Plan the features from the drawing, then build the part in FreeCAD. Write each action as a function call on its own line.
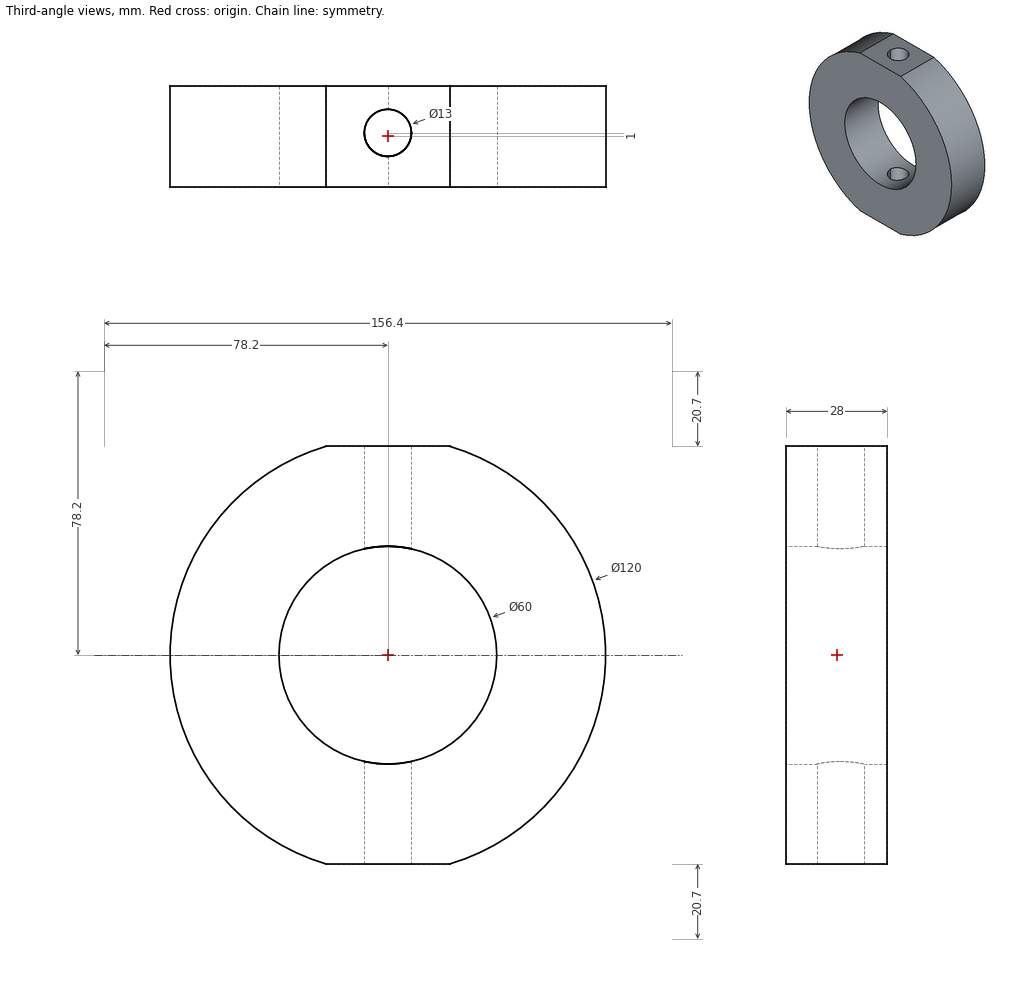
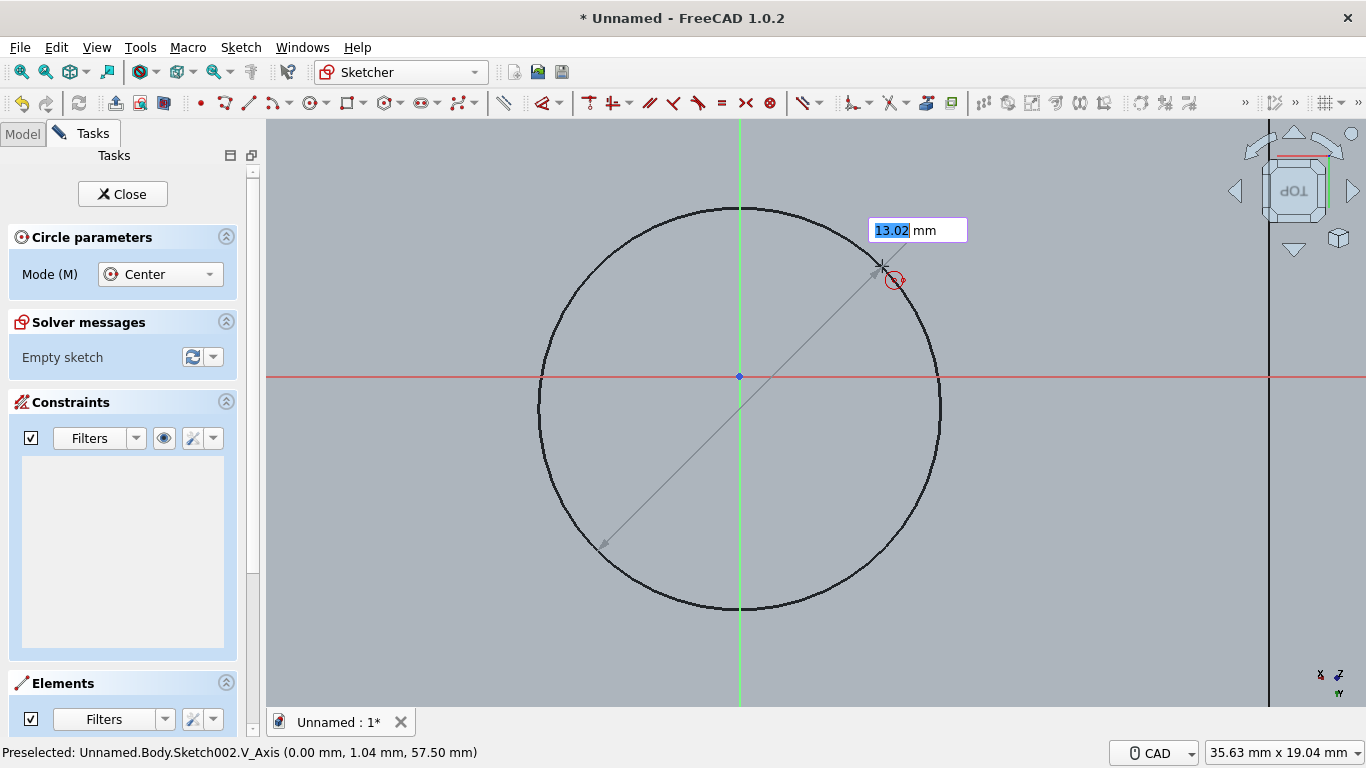
text(13)
key(Return)
key(Escape)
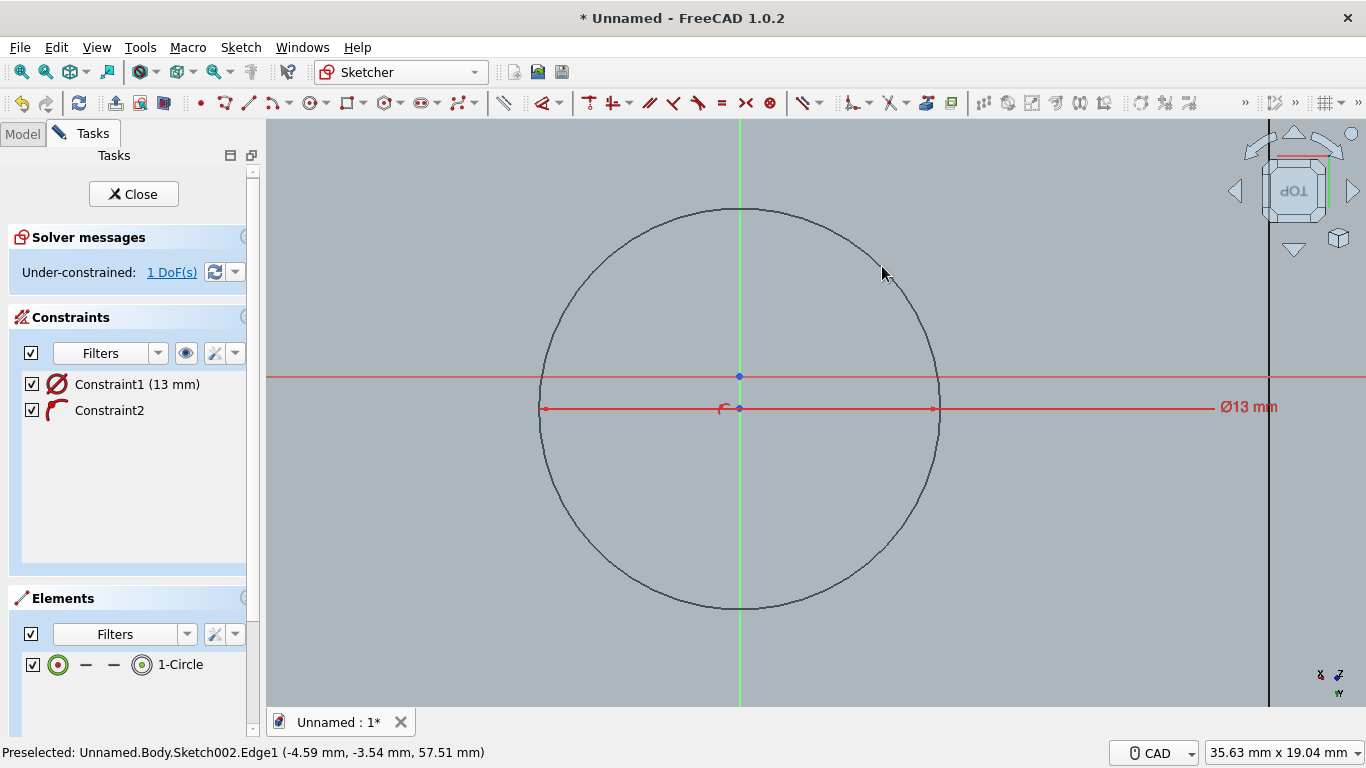
key(d)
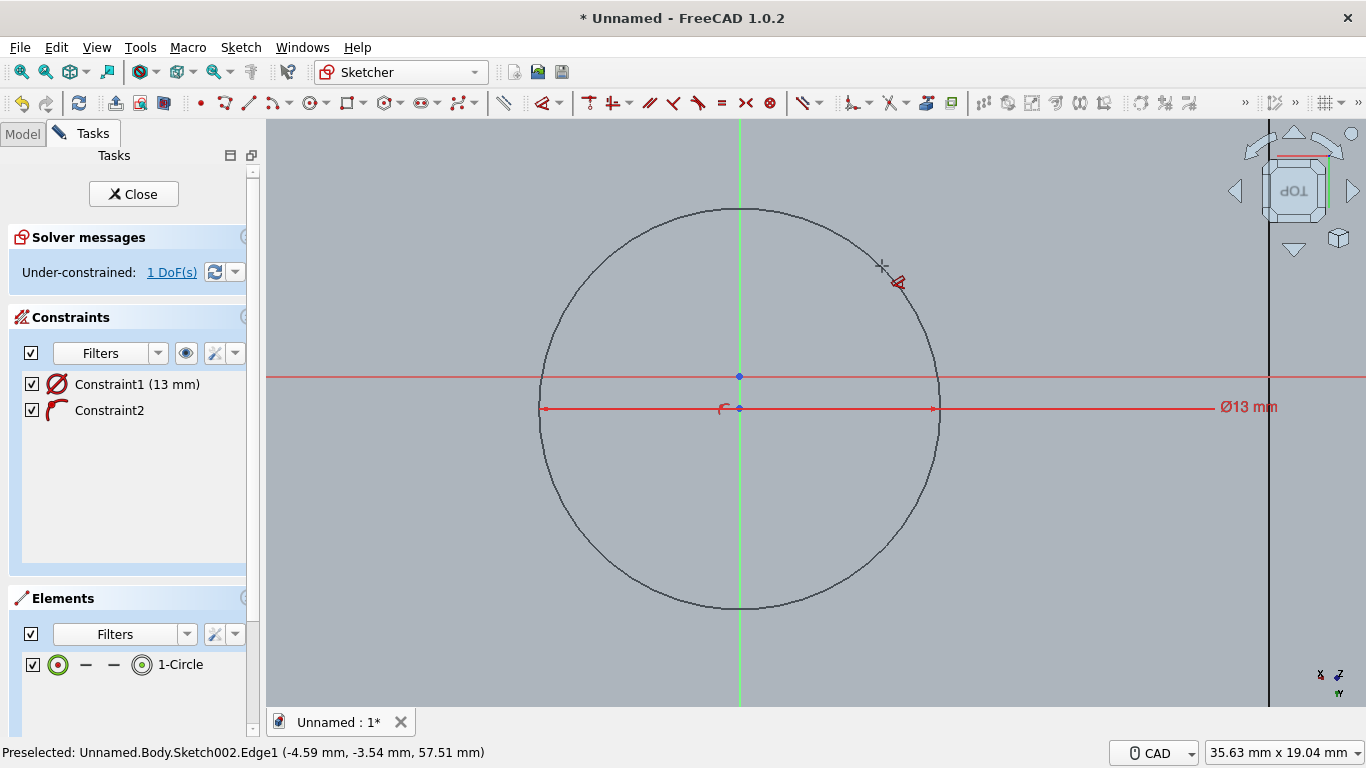
scroll(740, 409, up, 2)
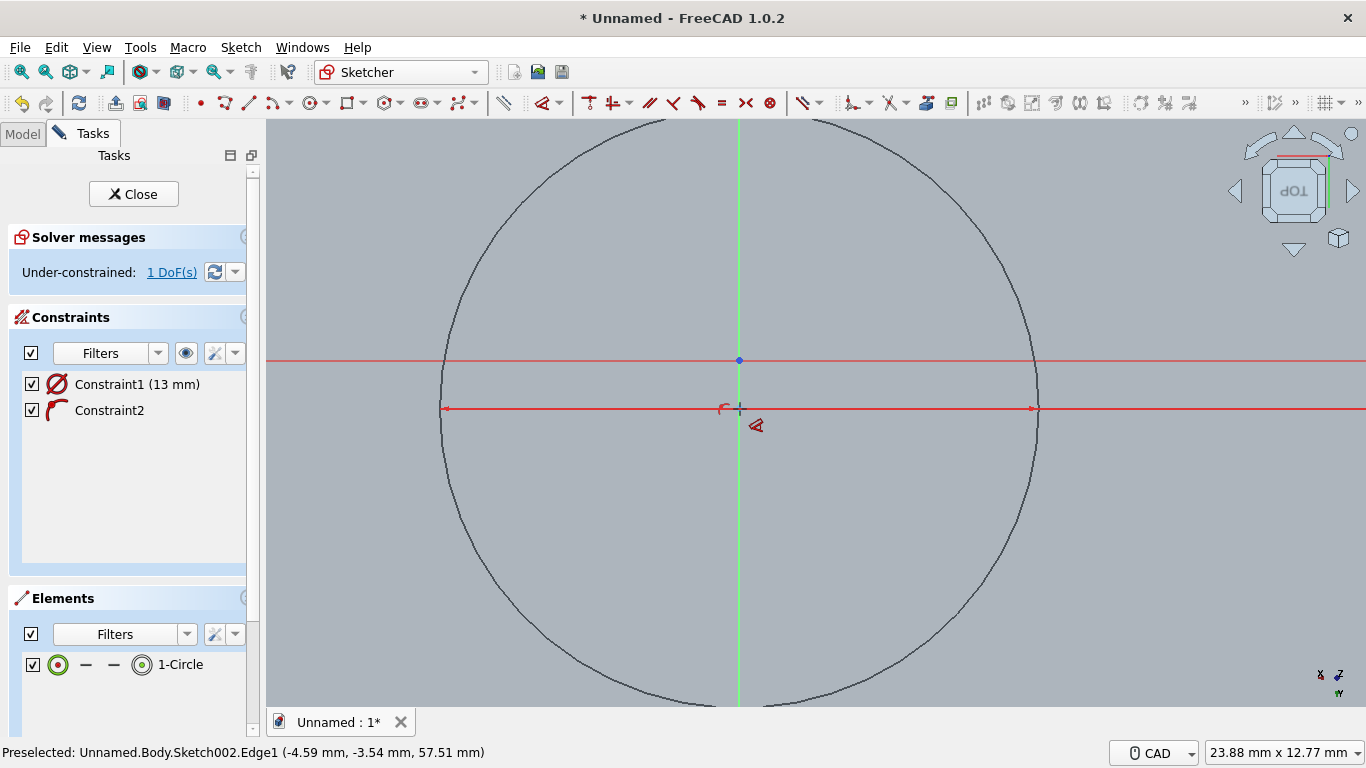
click(739, 409)
click(773, 385)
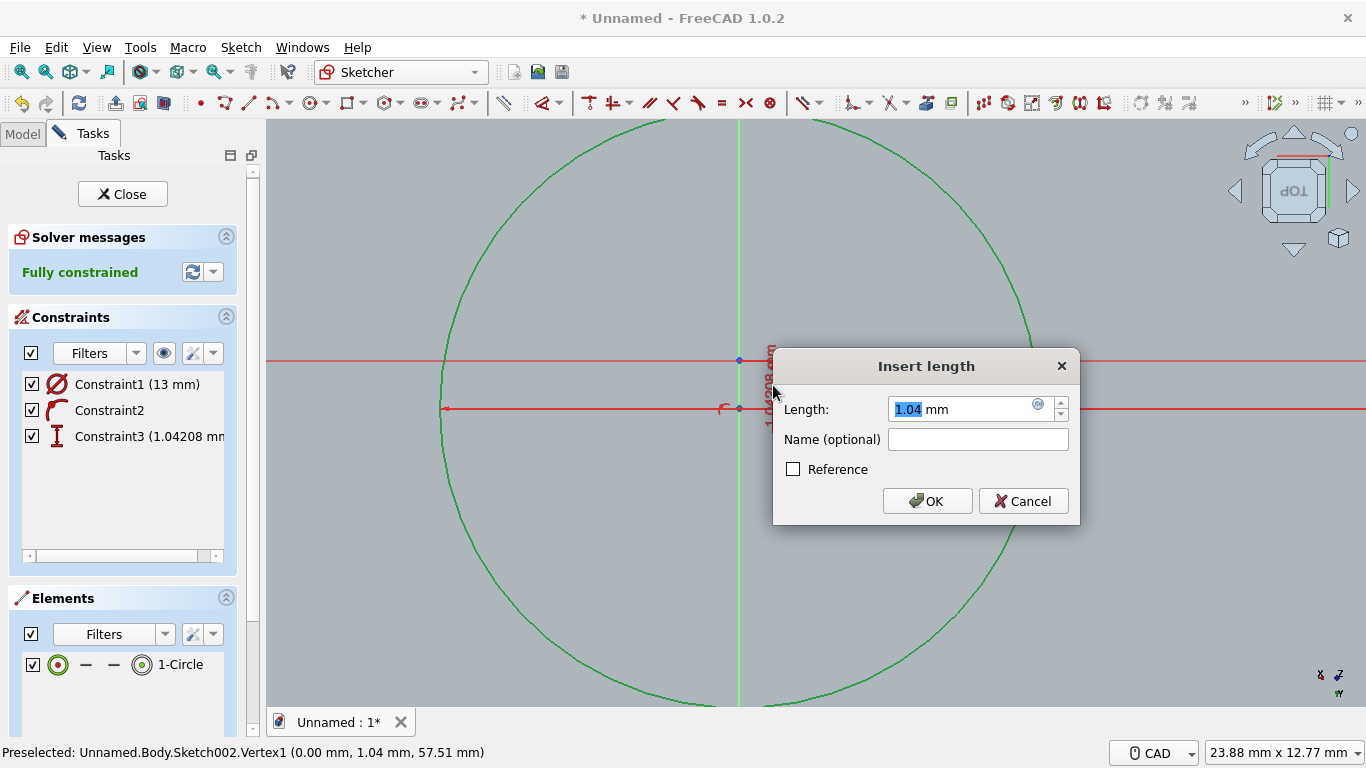
text(1)
key(Return)
key(Escape)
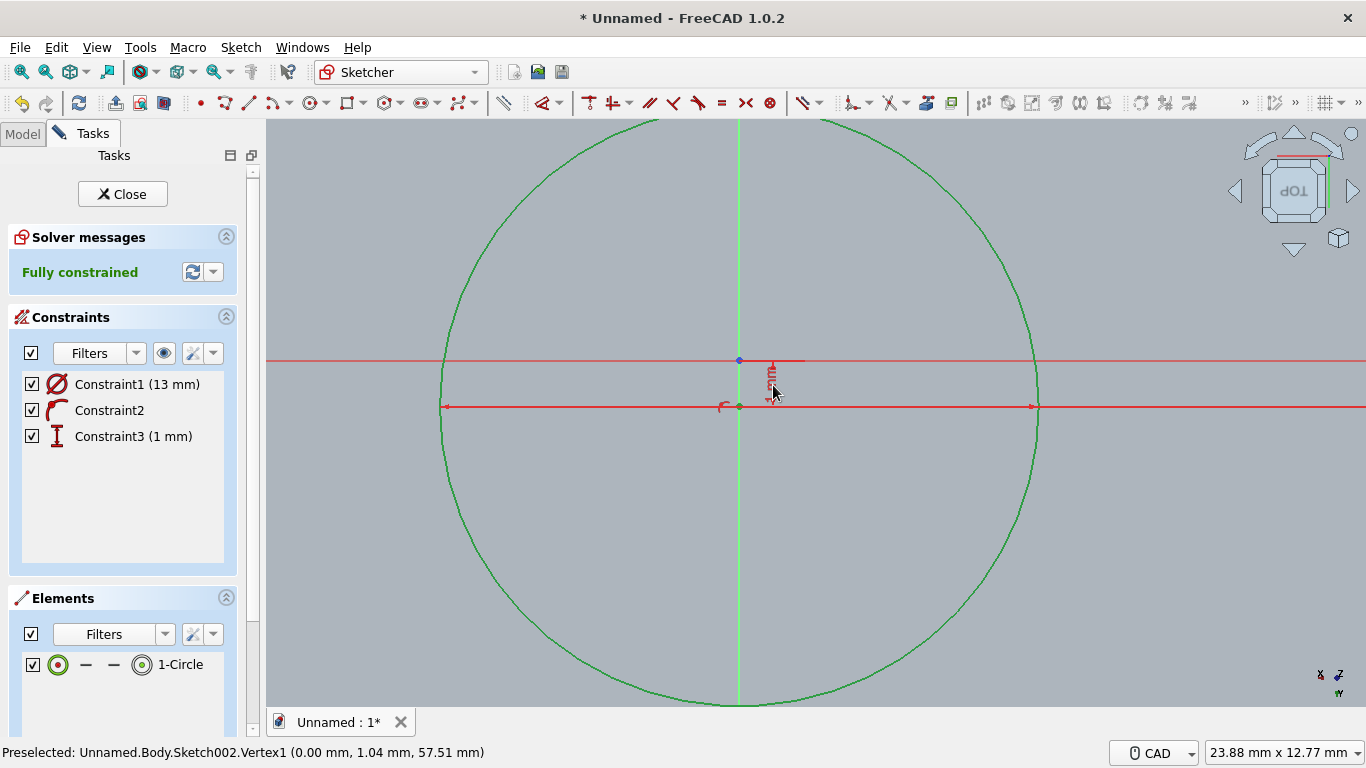
click(123, 194)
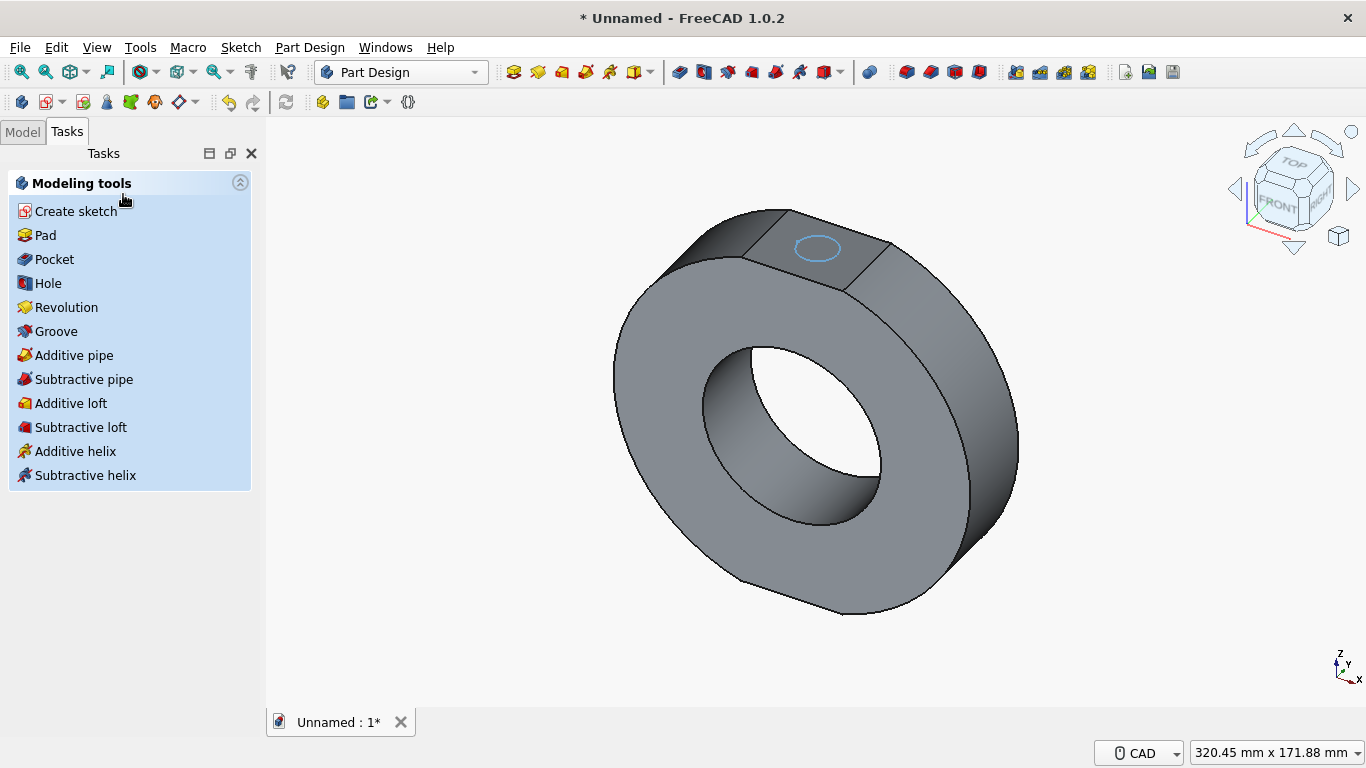
click(680, 72)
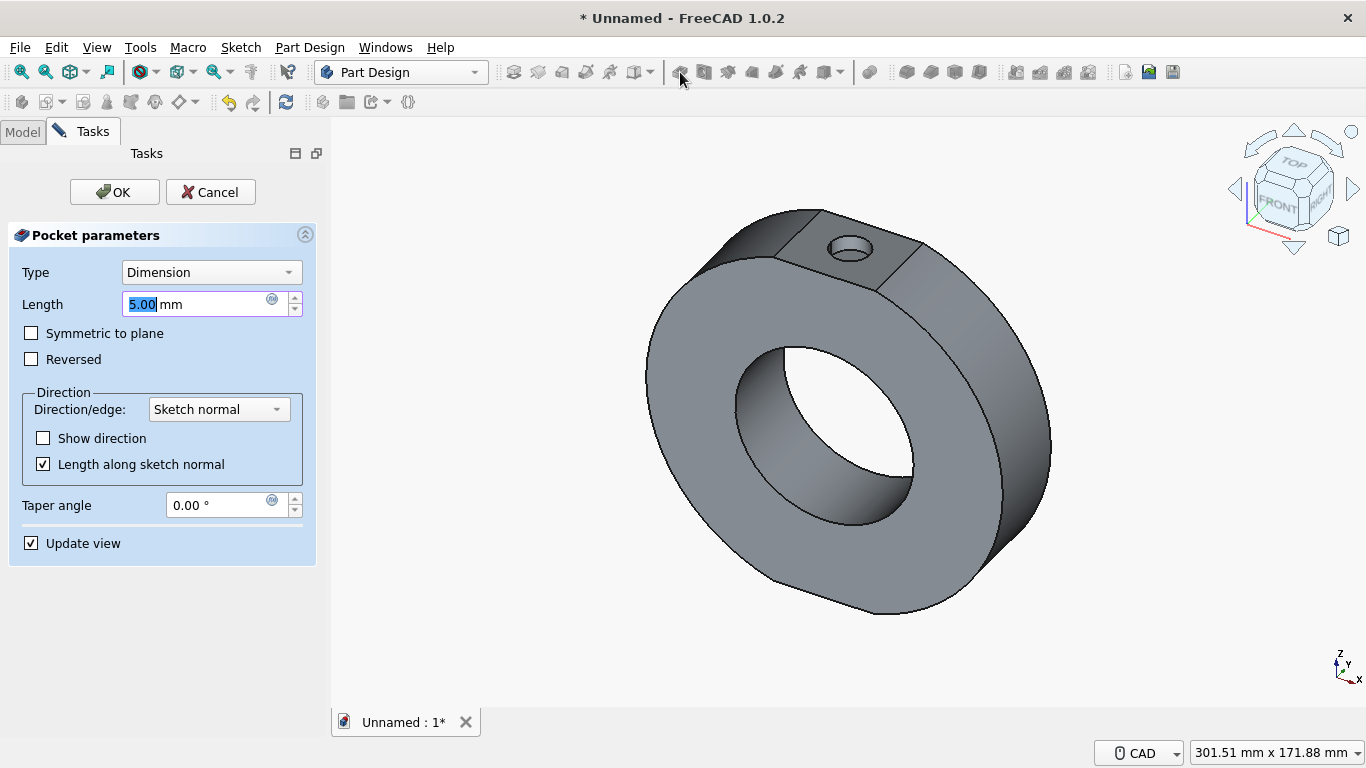
click(212, 272)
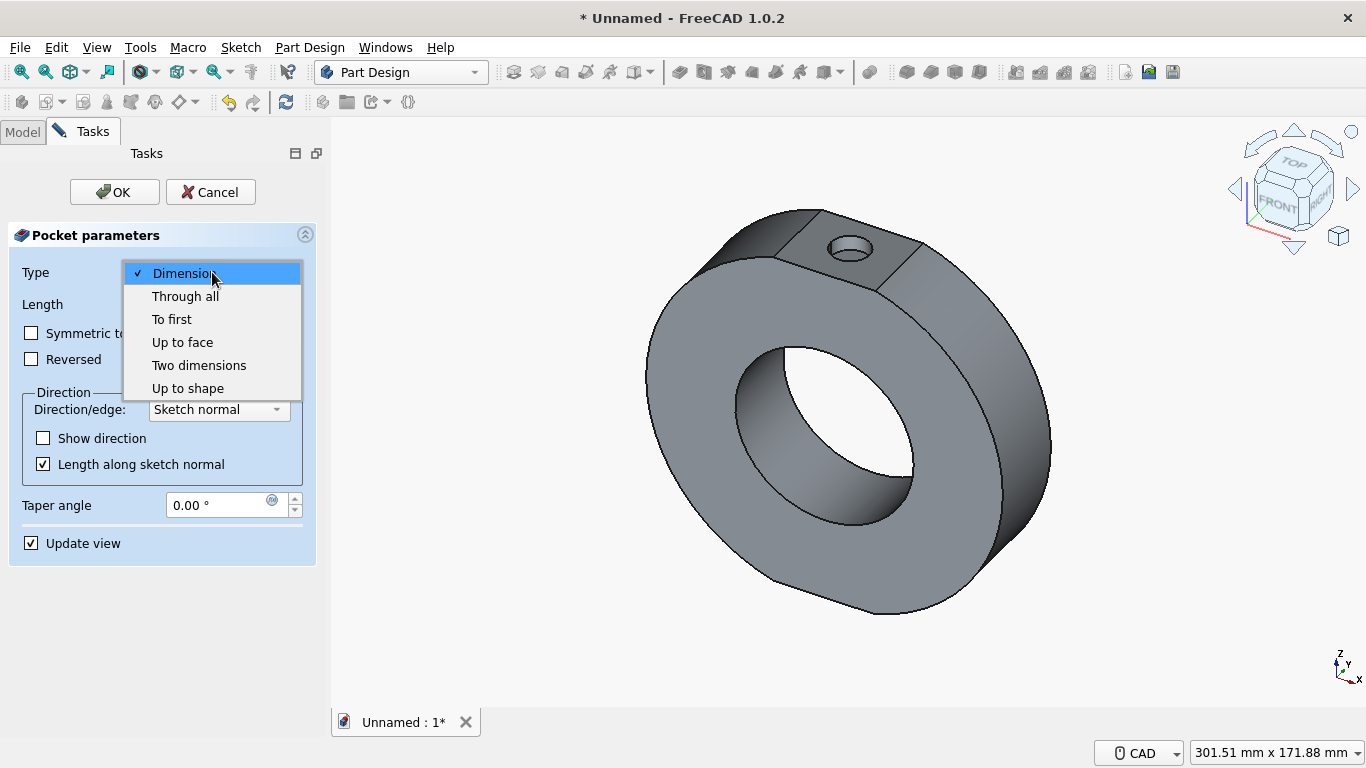
click(212, 296)